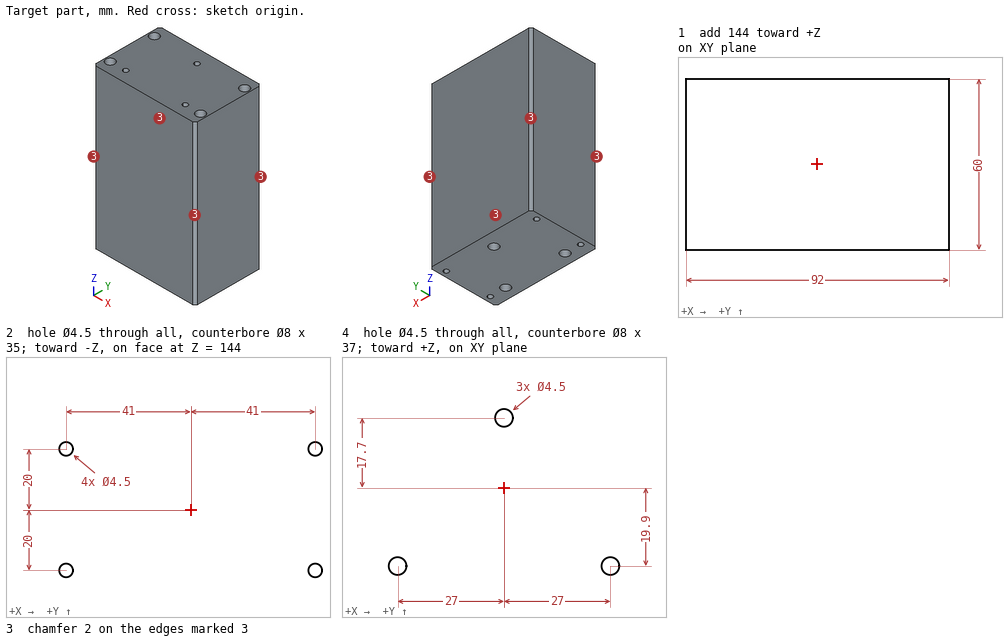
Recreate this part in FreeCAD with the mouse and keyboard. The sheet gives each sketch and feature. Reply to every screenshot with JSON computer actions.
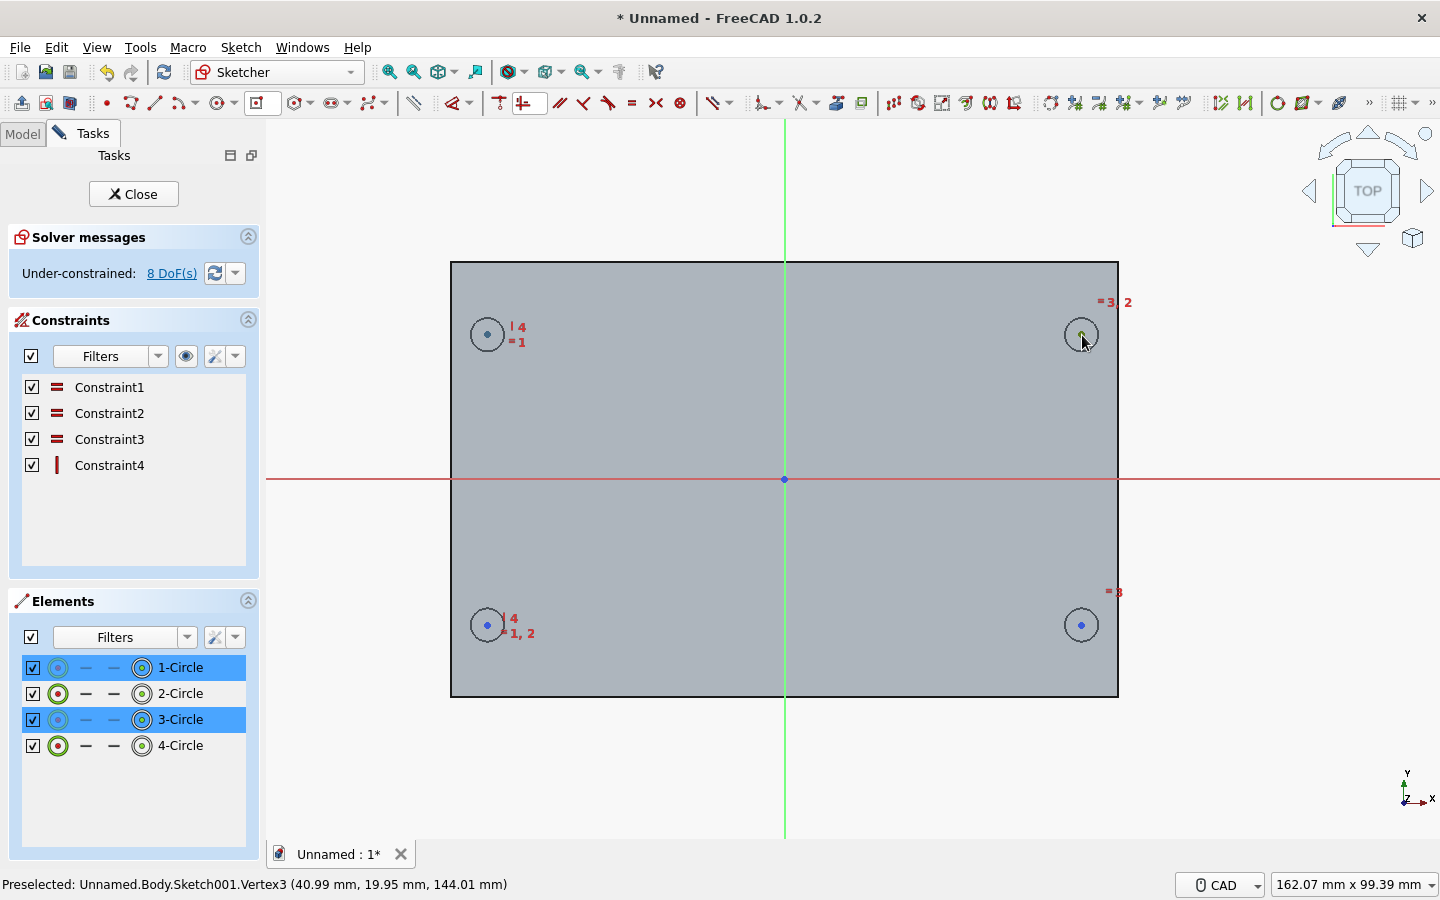
{"action": "left_click", "coordinate": [542, 104]}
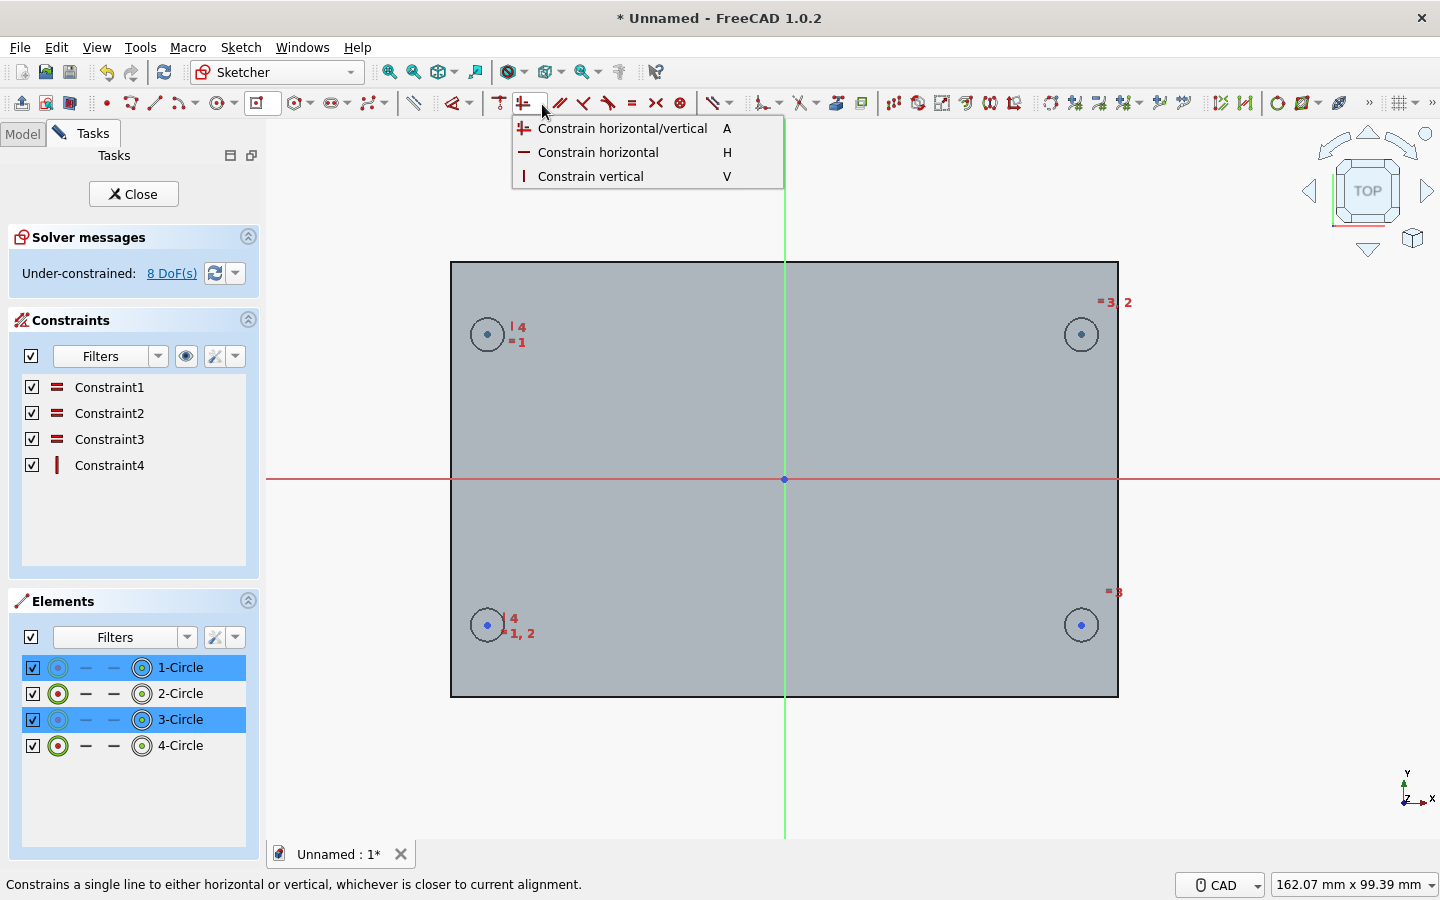
{"action": "left_click", "coordinate": [648, 152]}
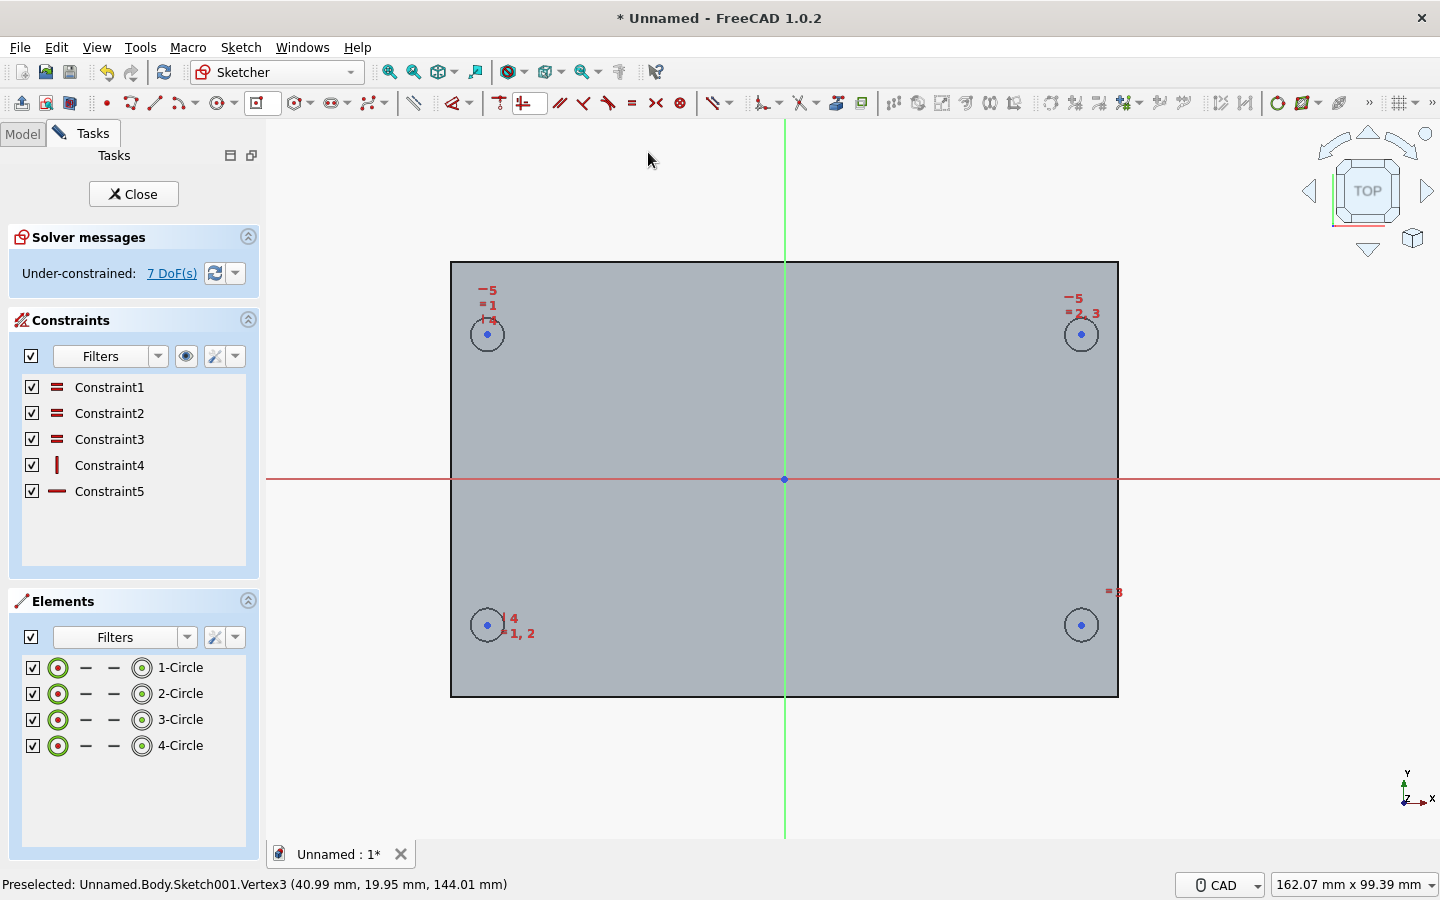
{"action": "left_click", "coordinate": [1082, 335]}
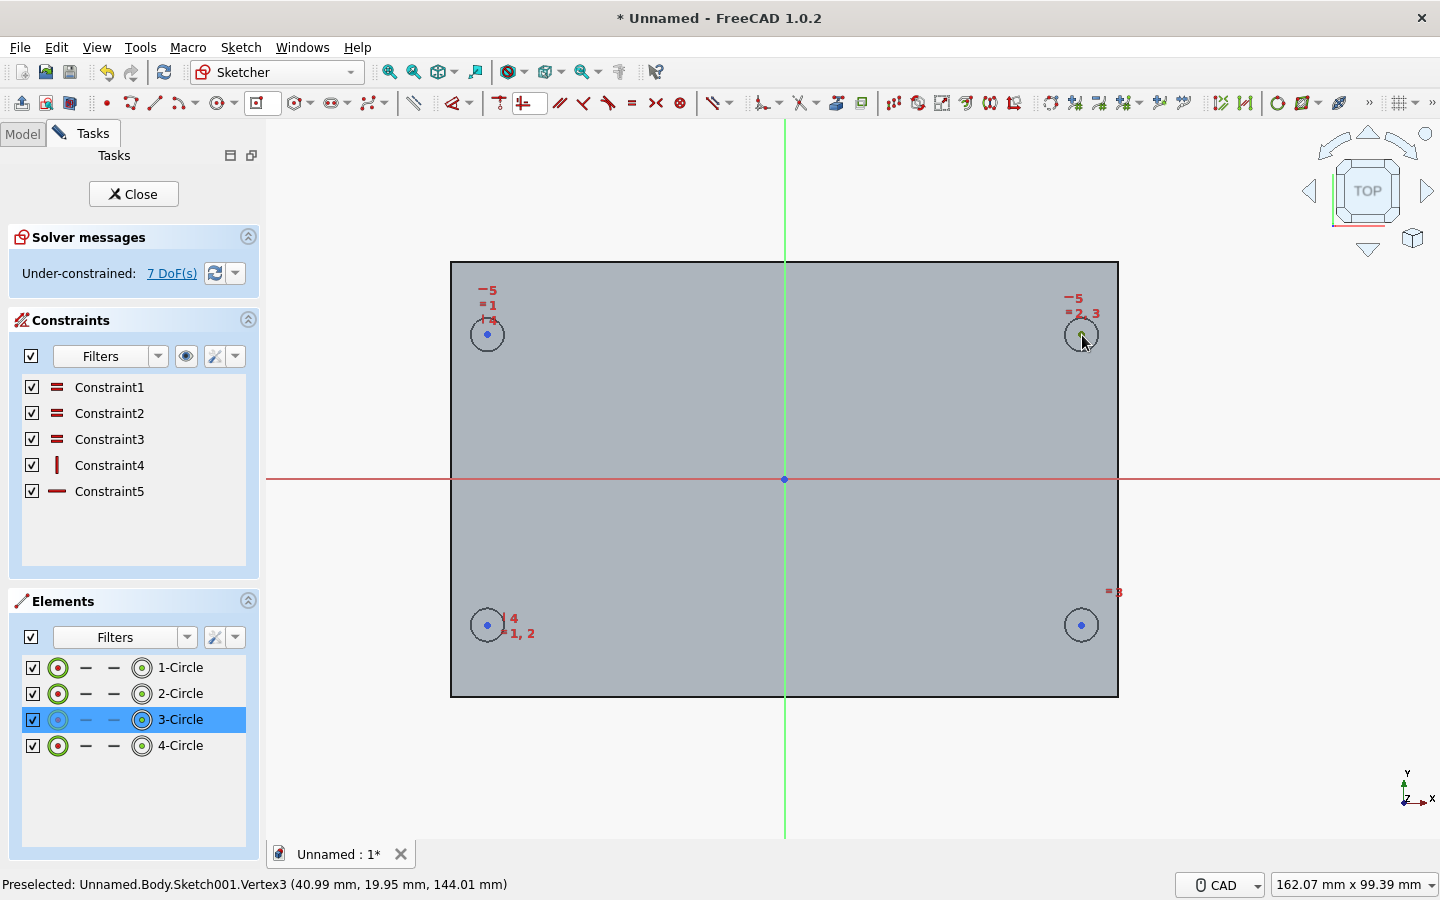
{"action": "left_click", "coordinate": [1082, 625]}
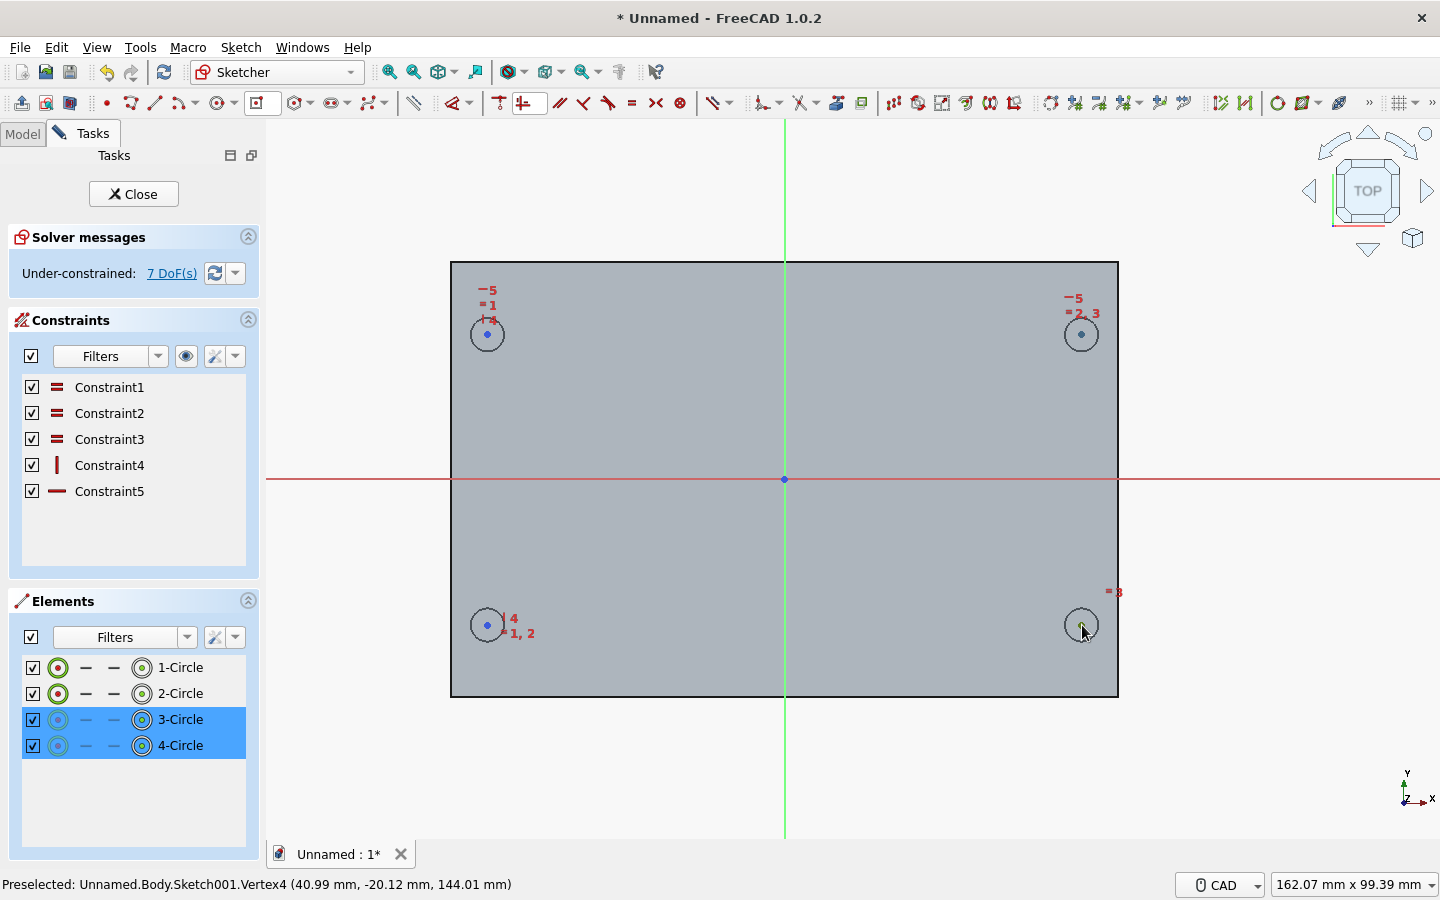
{"action": "left_click", "coordinate": [542, 104]}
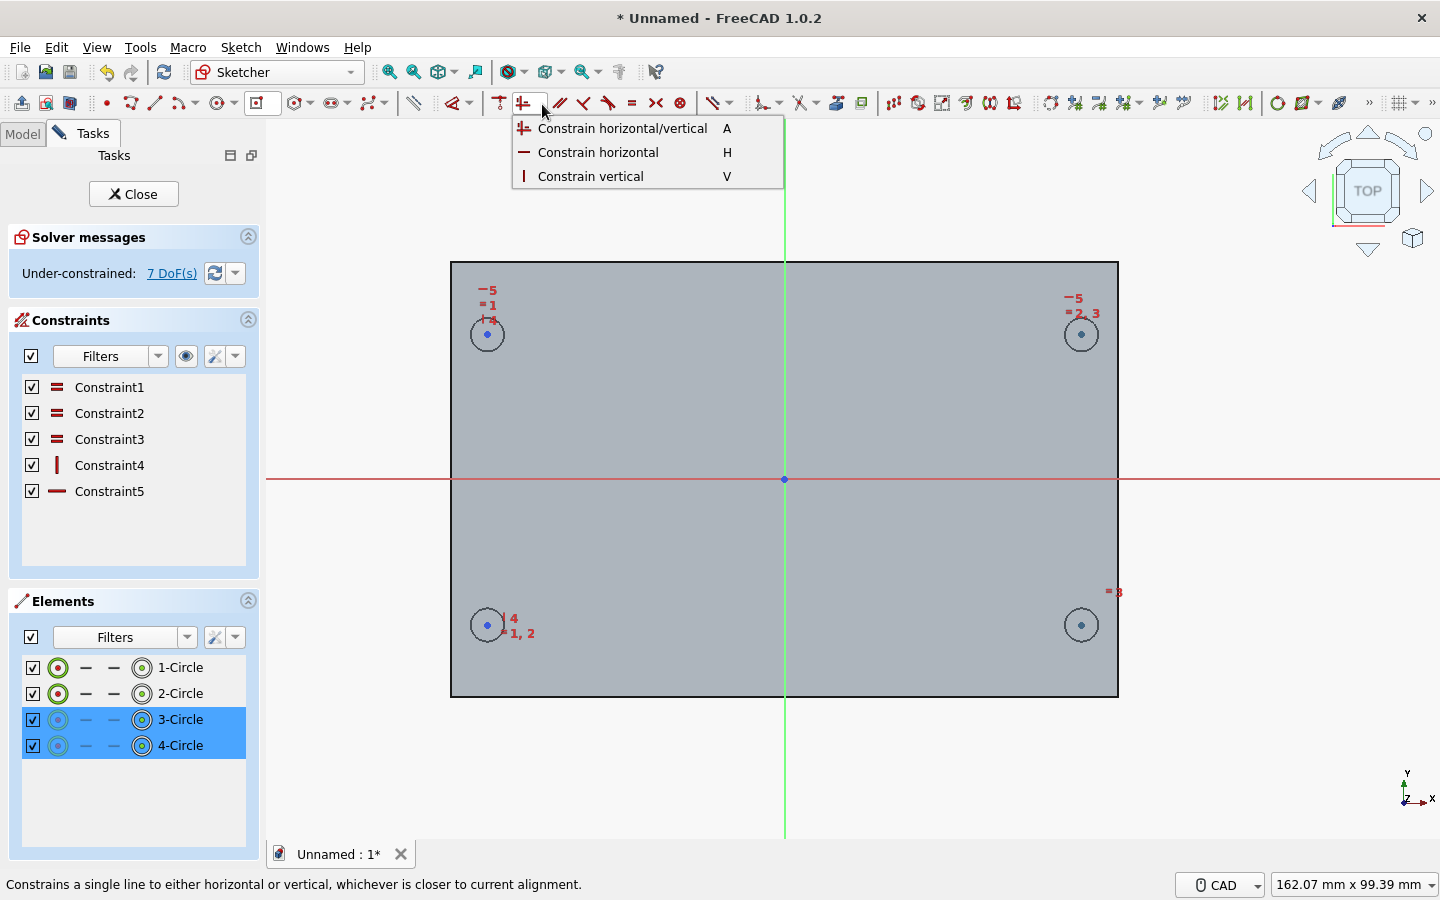
{"action": "left_click", "coordinate": [648, 176]}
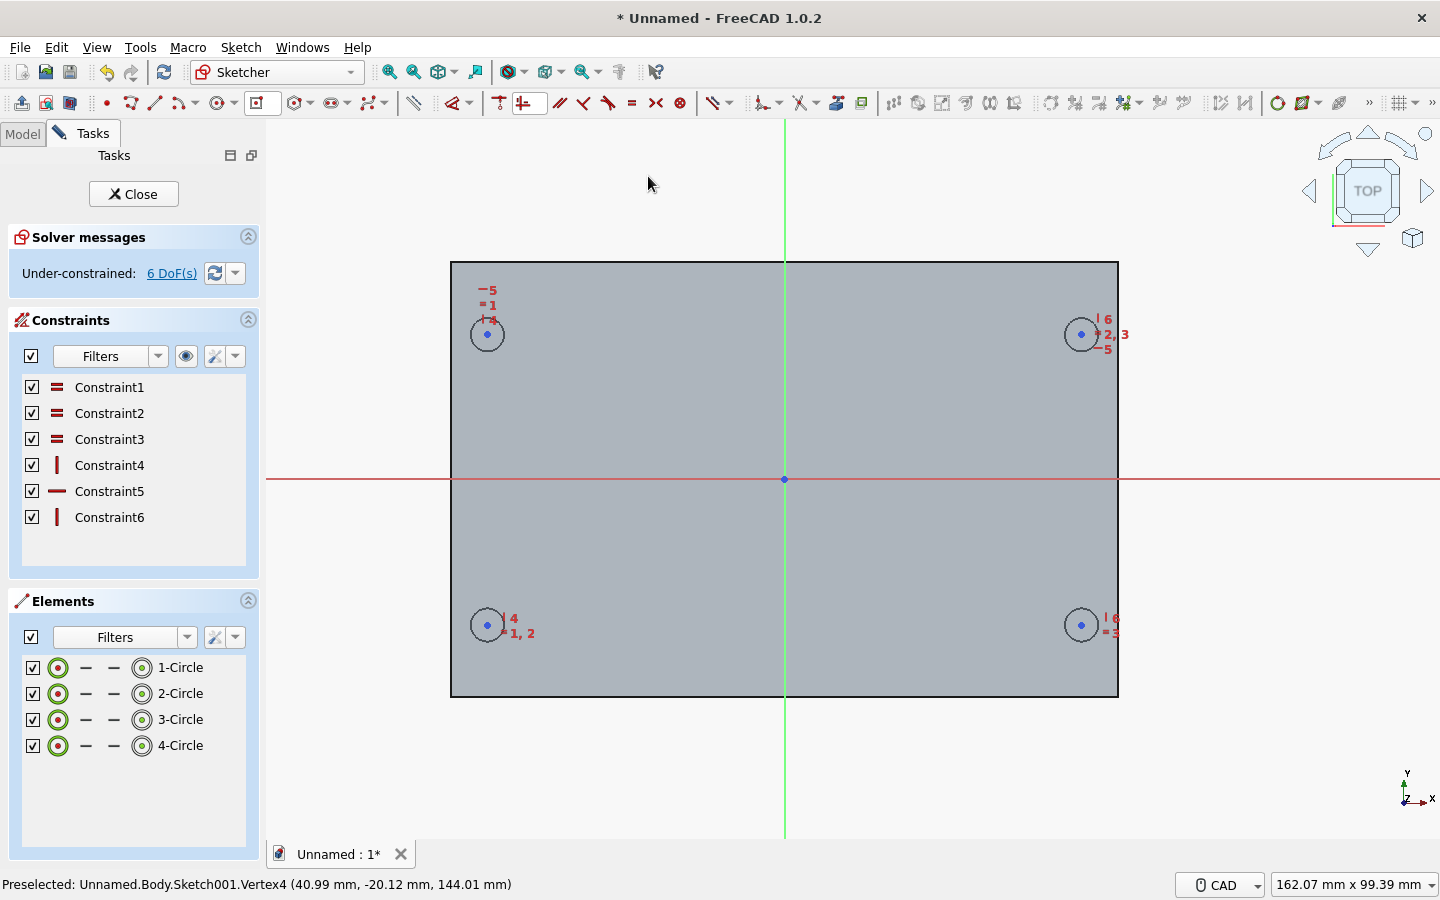
{"action": "left_click", "coordinate": [487, 625]}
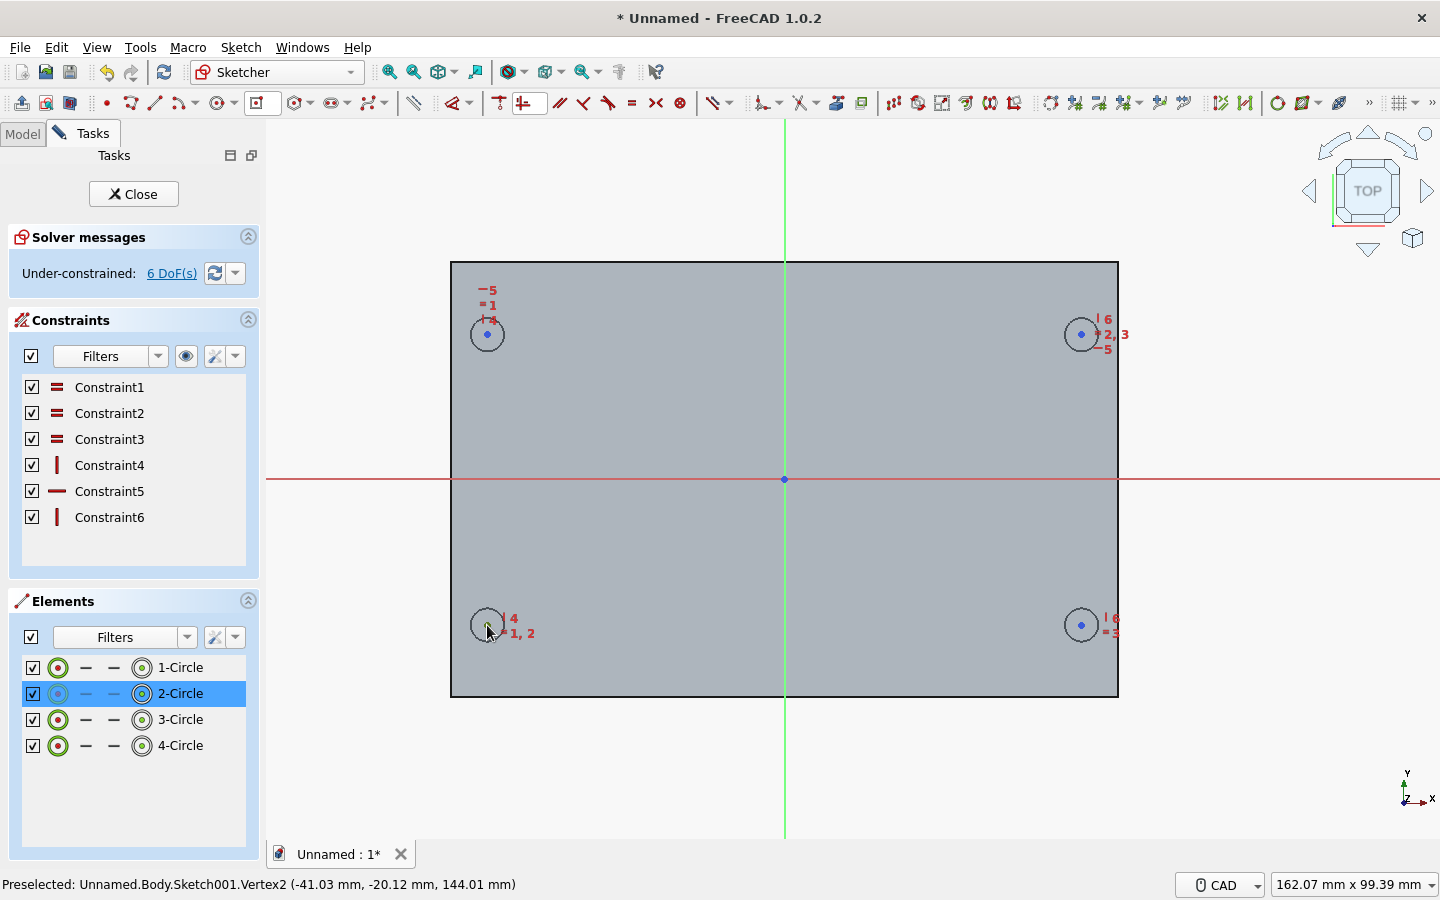
{"action": "left_click", "coordinate": [1082, 625]}